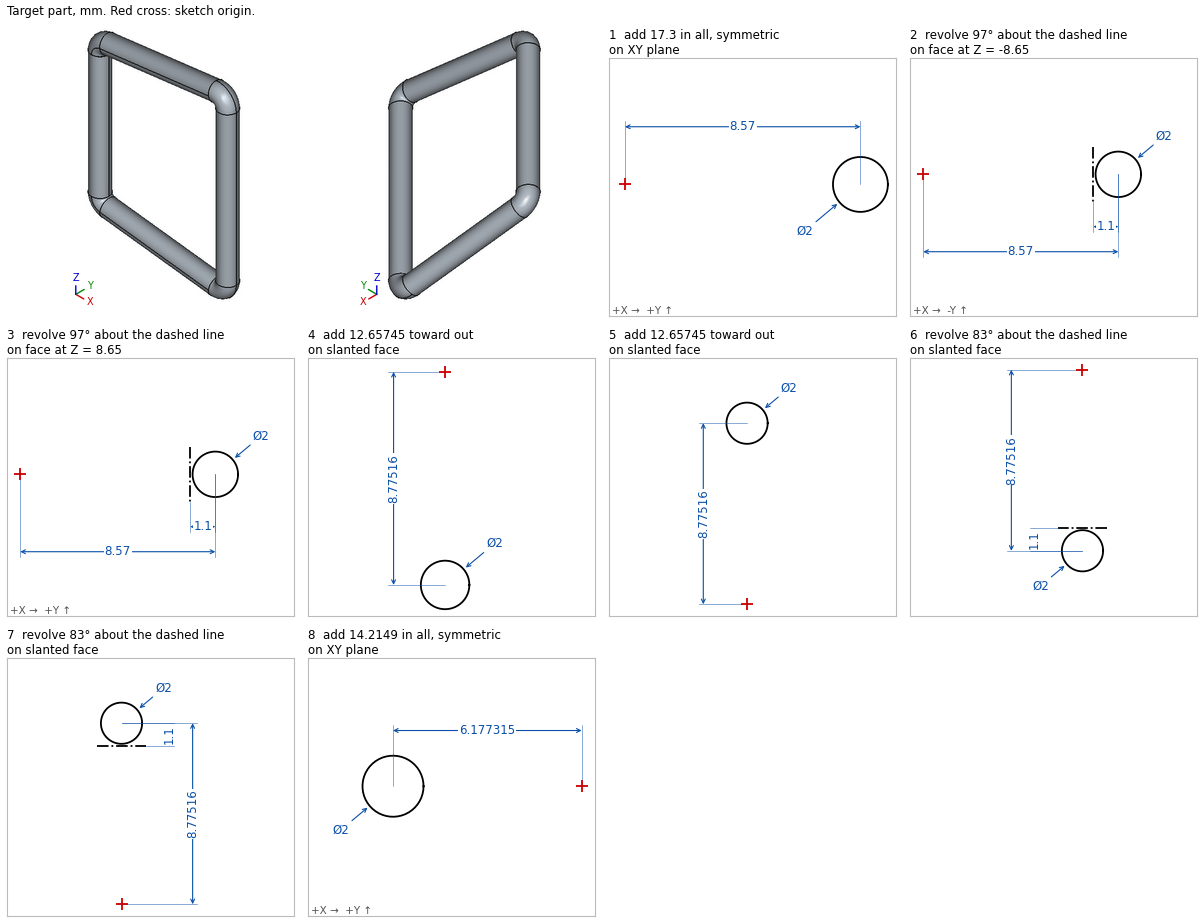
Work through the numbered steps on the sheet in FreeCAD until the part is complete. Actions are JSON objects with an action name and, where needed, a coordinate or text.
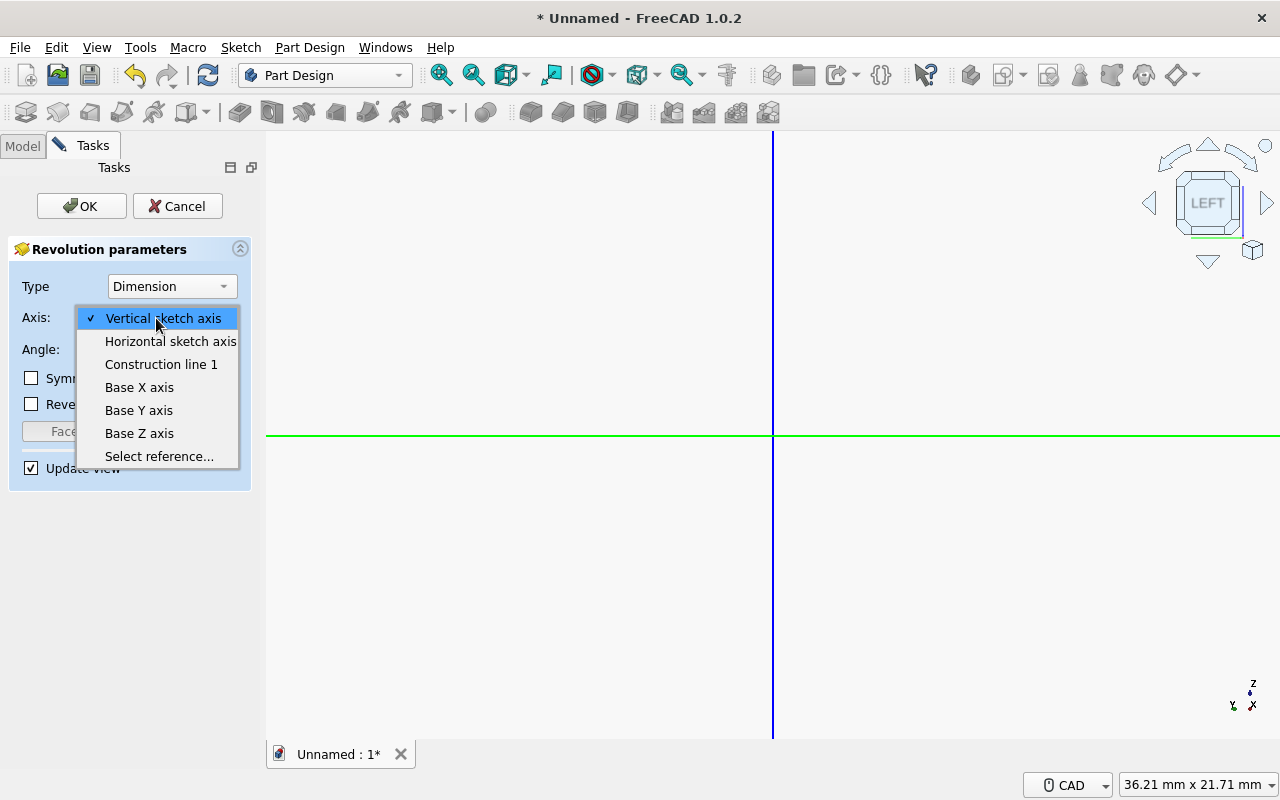
{"action": "left_click", "coordinate": [156, 364]}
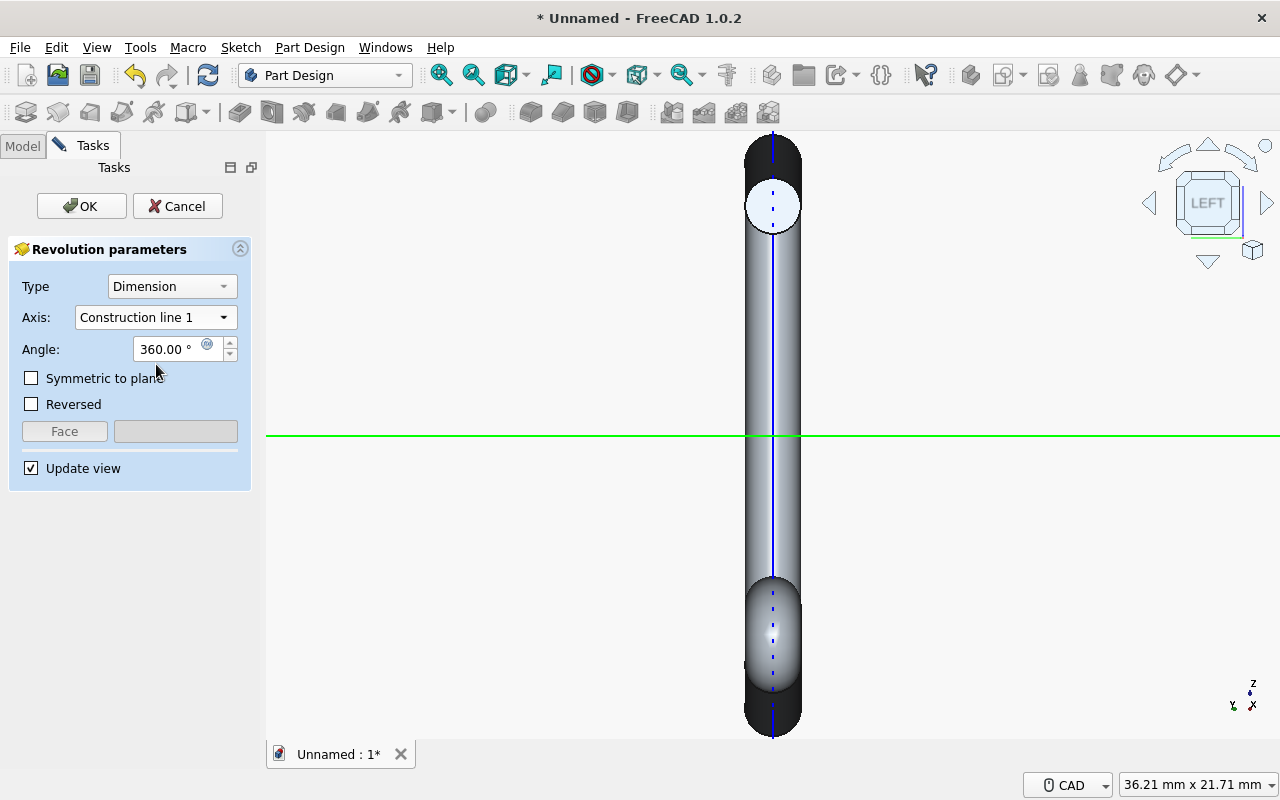
{"action": "triple_click", "coordinate": [178, 349]}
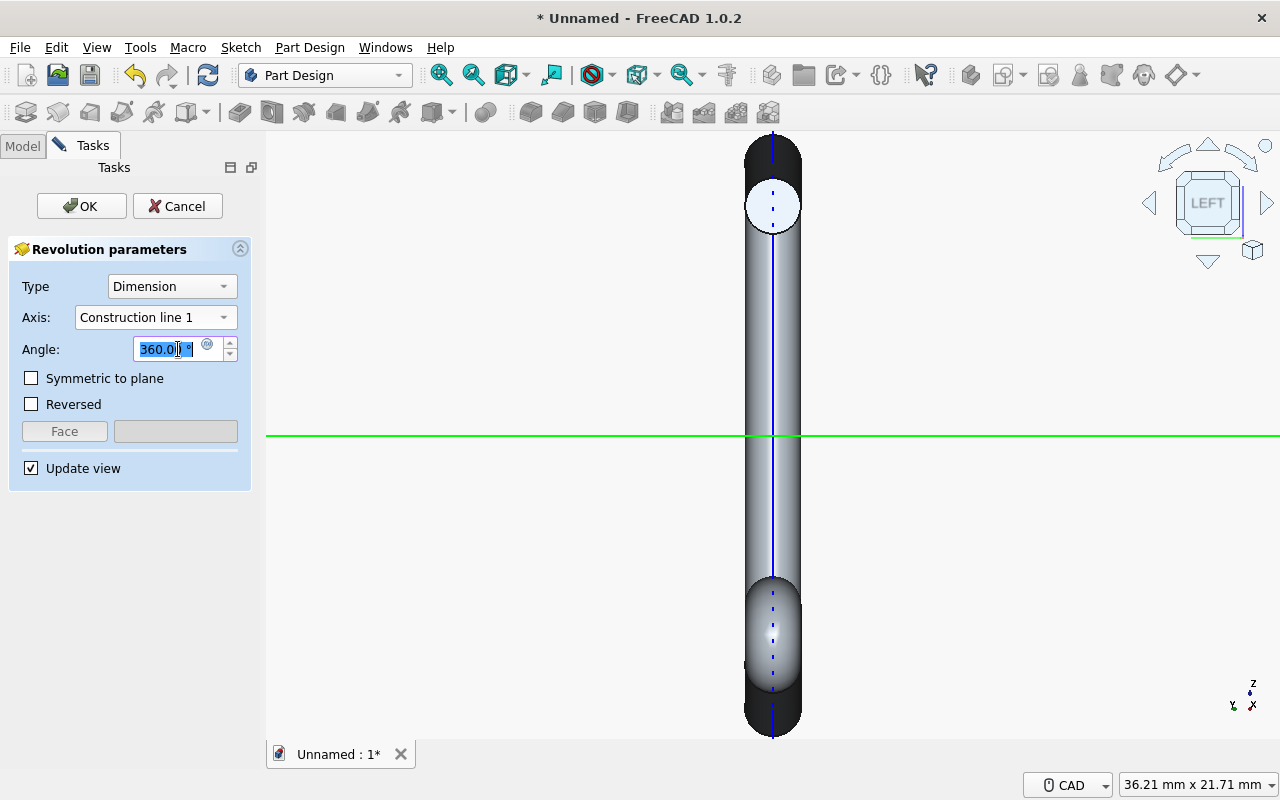
{"action": "type", "text": "83"}
{"action": "key", "text": "Tab"}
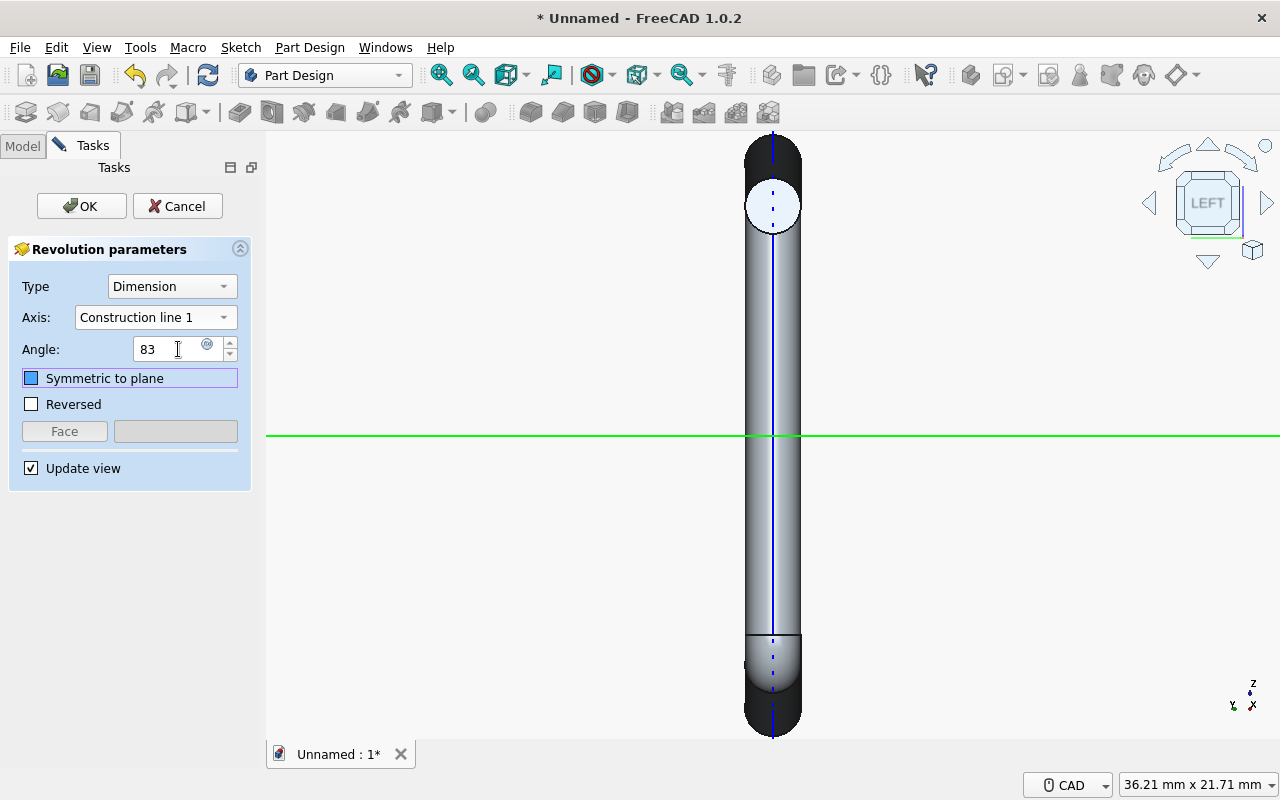
{"action": "left_click", "coordinate": [82, 206]}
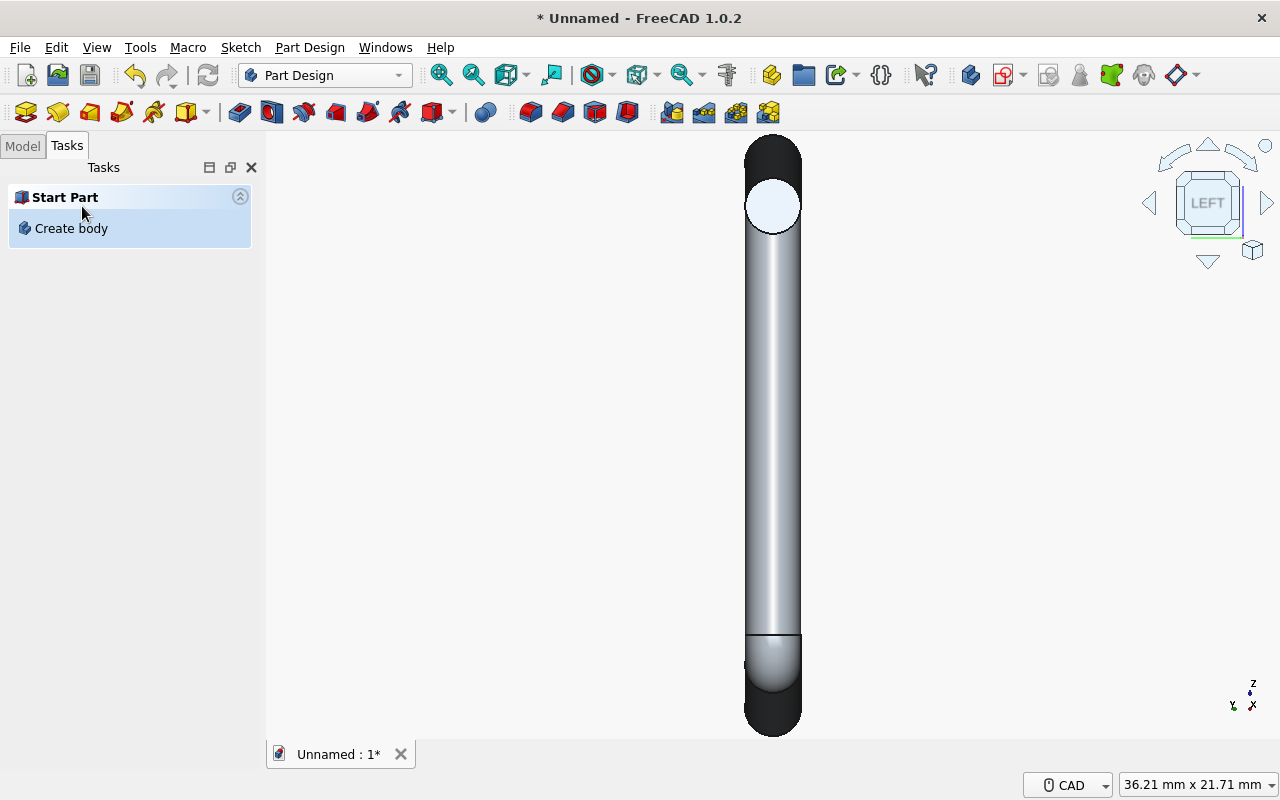
{"action": "left_click", "coordinate": [773, 205]}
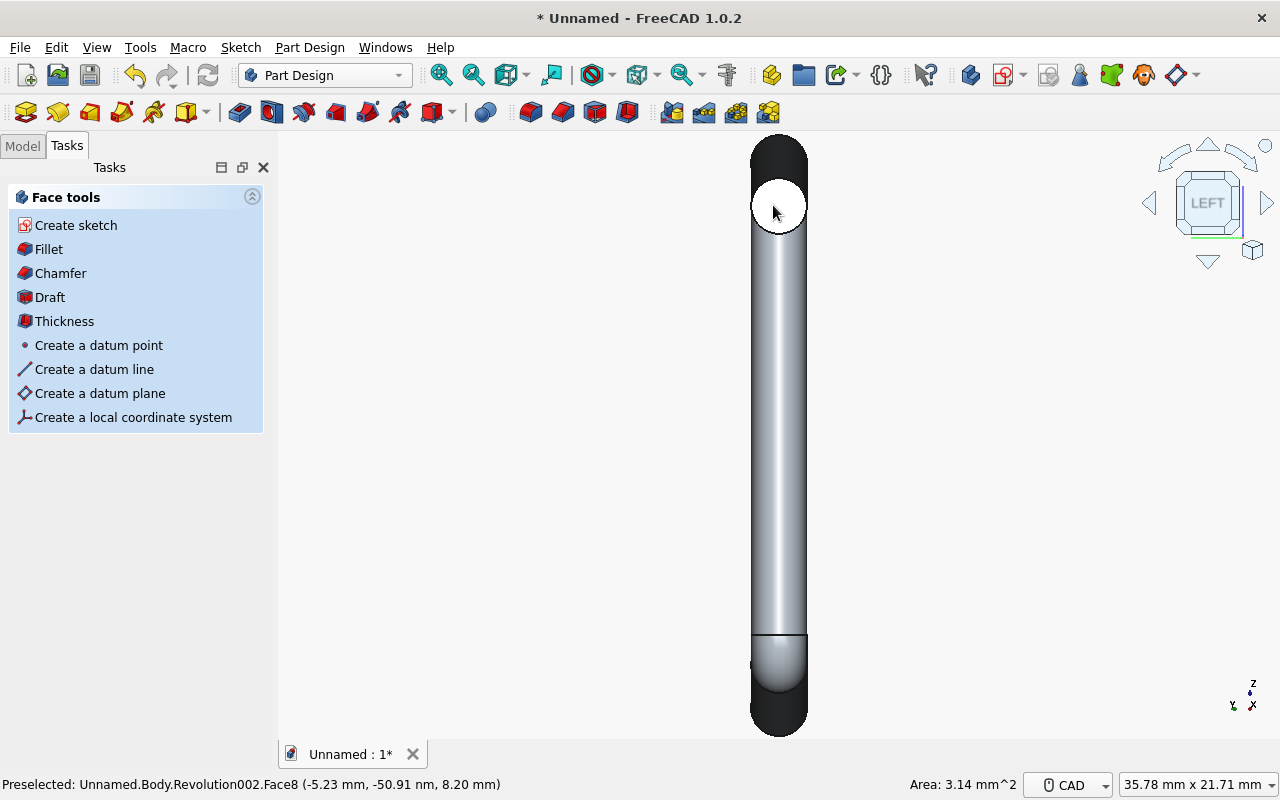
{"action": "left_click", "coordinate": [1004, 76]}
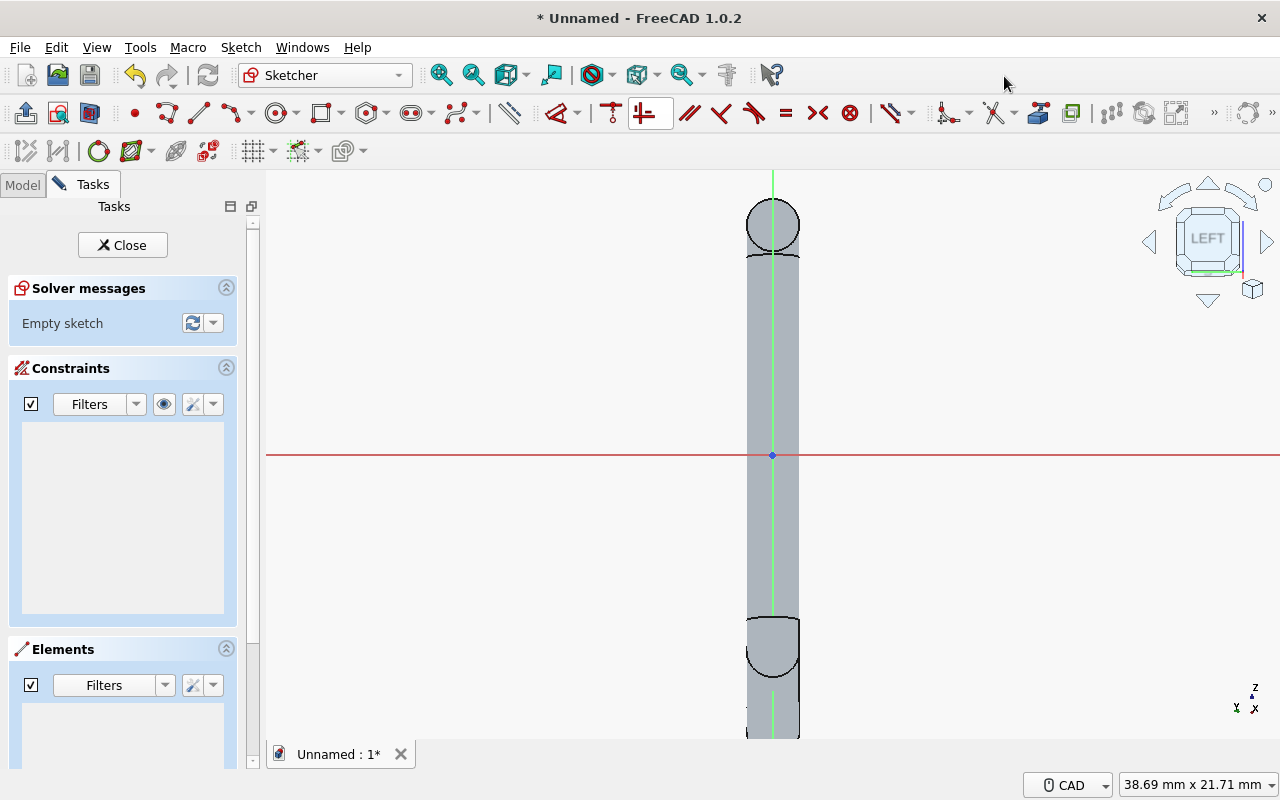
{"action": "scroll", "coordinate": [704, 454], "scroll_direction": "down", "scroll_amount": 5}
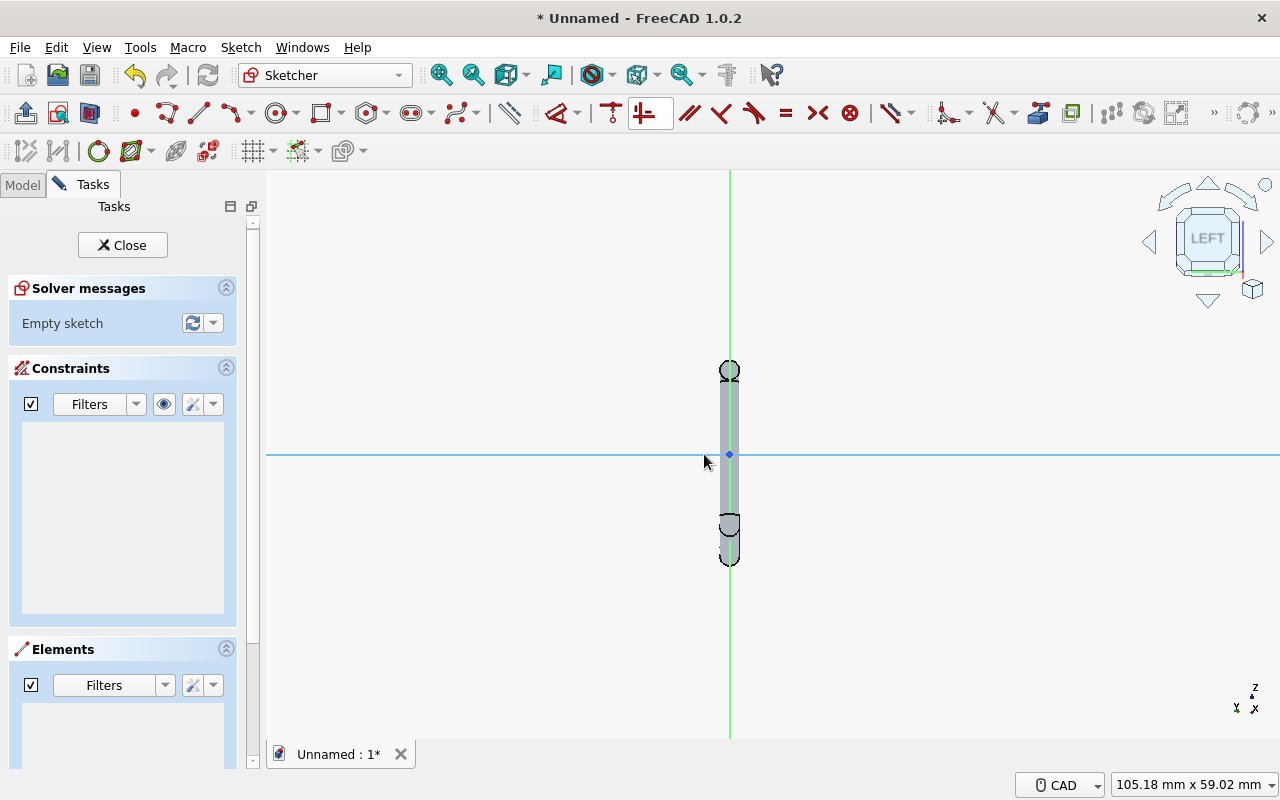
{"action": "scroll", "coordinate": [731, 365], "scroll_direction": "up", "scroll_amount": 14}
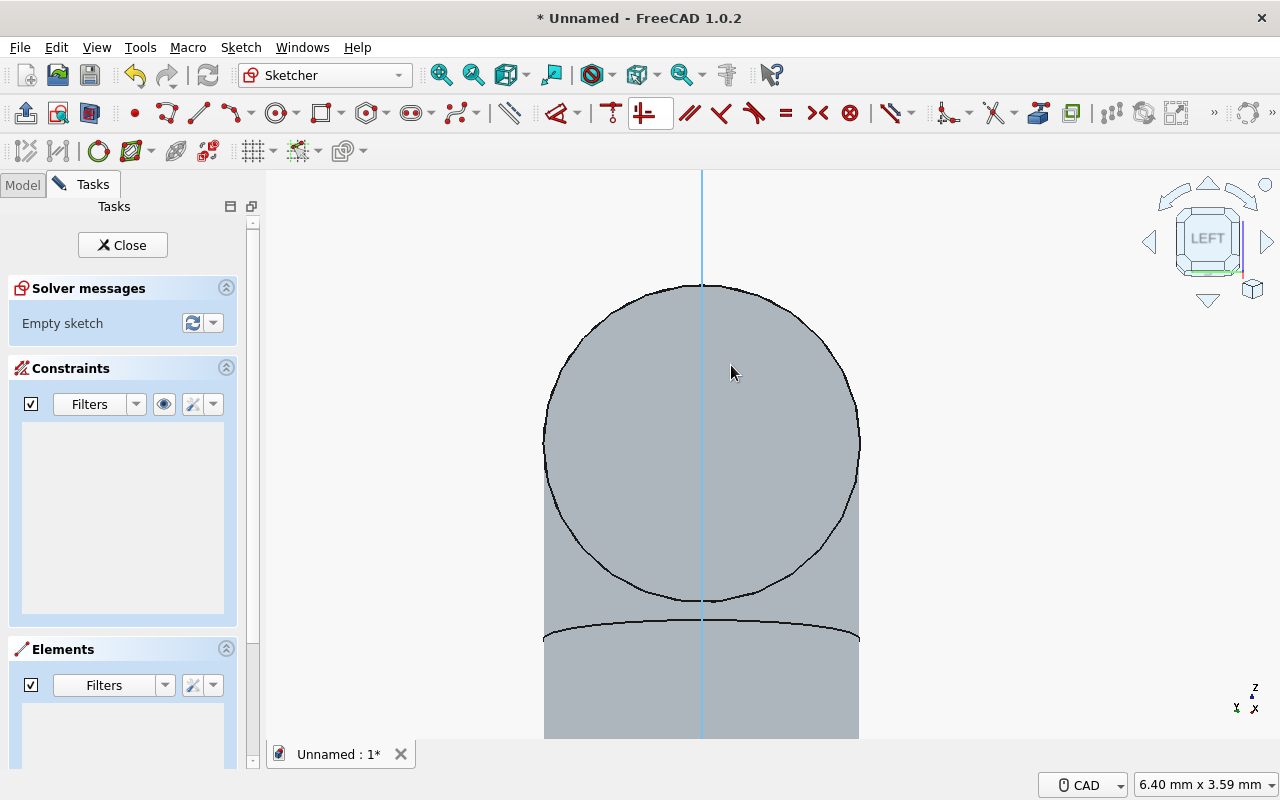
{"action": "left_click", "coordinate": [276, 114]}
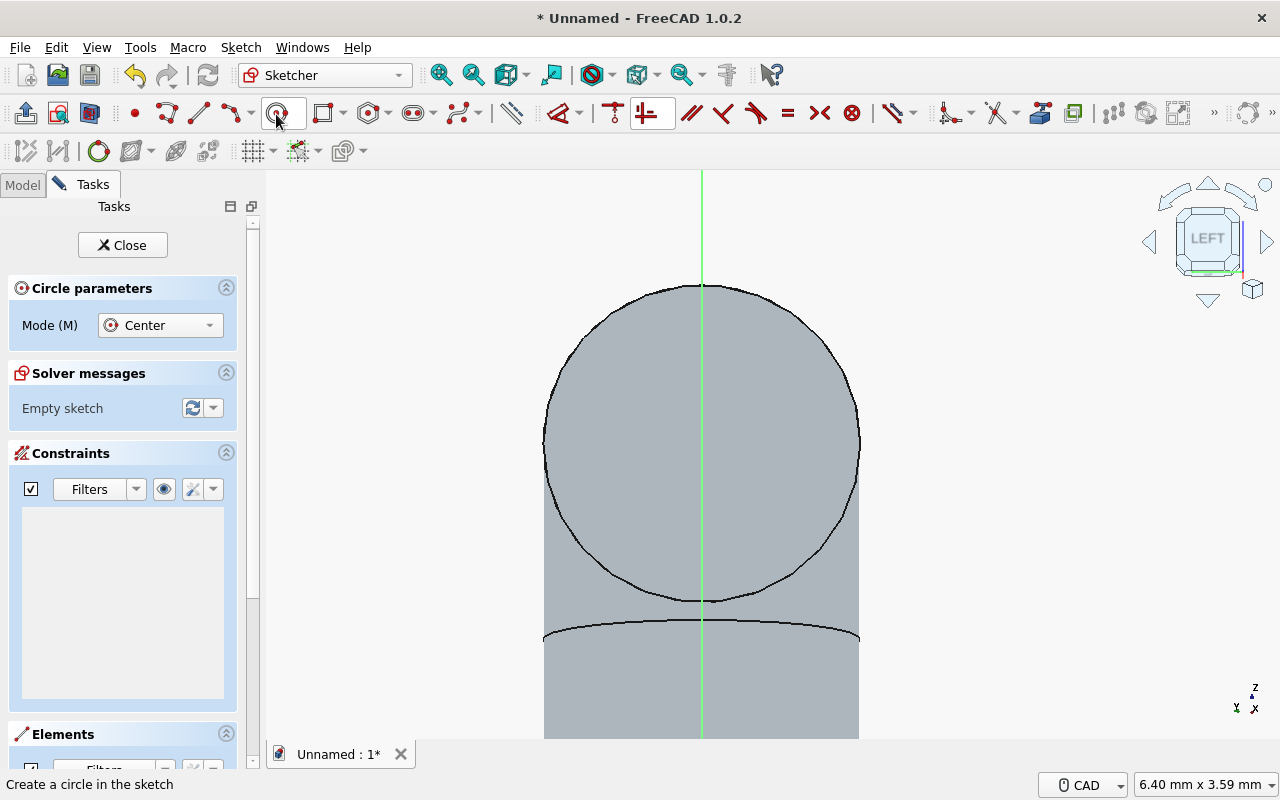
{"action": "left_click", "coordinate": [702, 444]}
{"action": "mouse_move", "coordinate": [814, 332]}